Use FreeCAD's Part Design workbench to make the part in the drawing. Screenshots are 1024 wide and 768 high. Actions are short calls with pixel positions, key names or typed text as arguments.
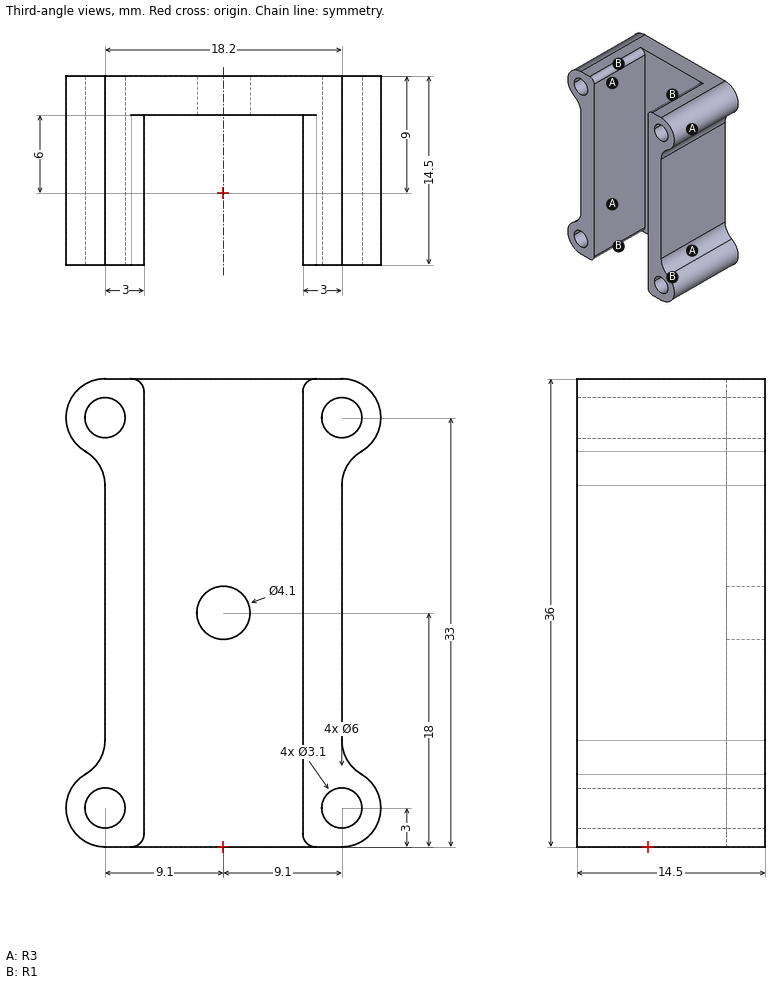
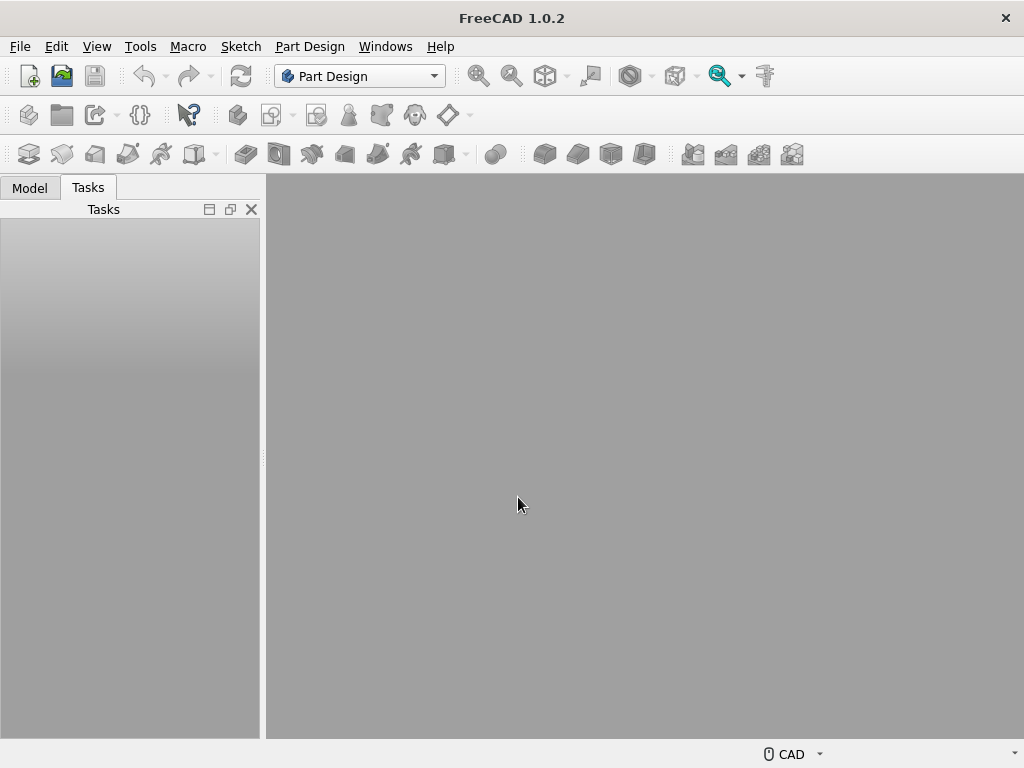
click(29, 76)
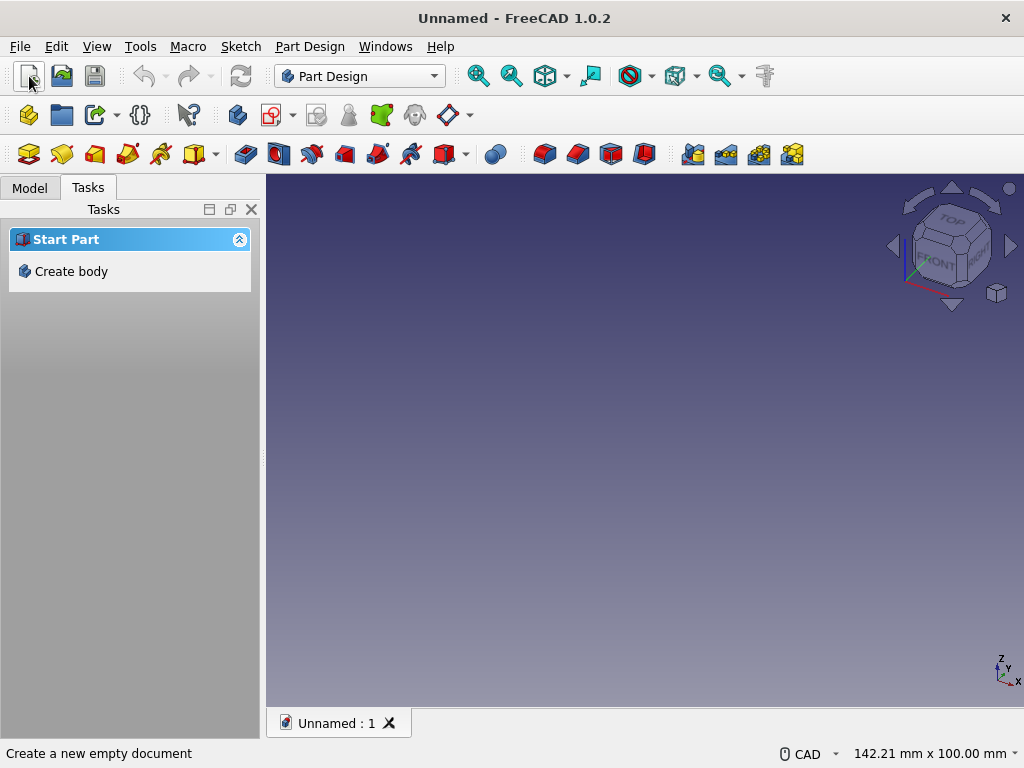
click(270, 116)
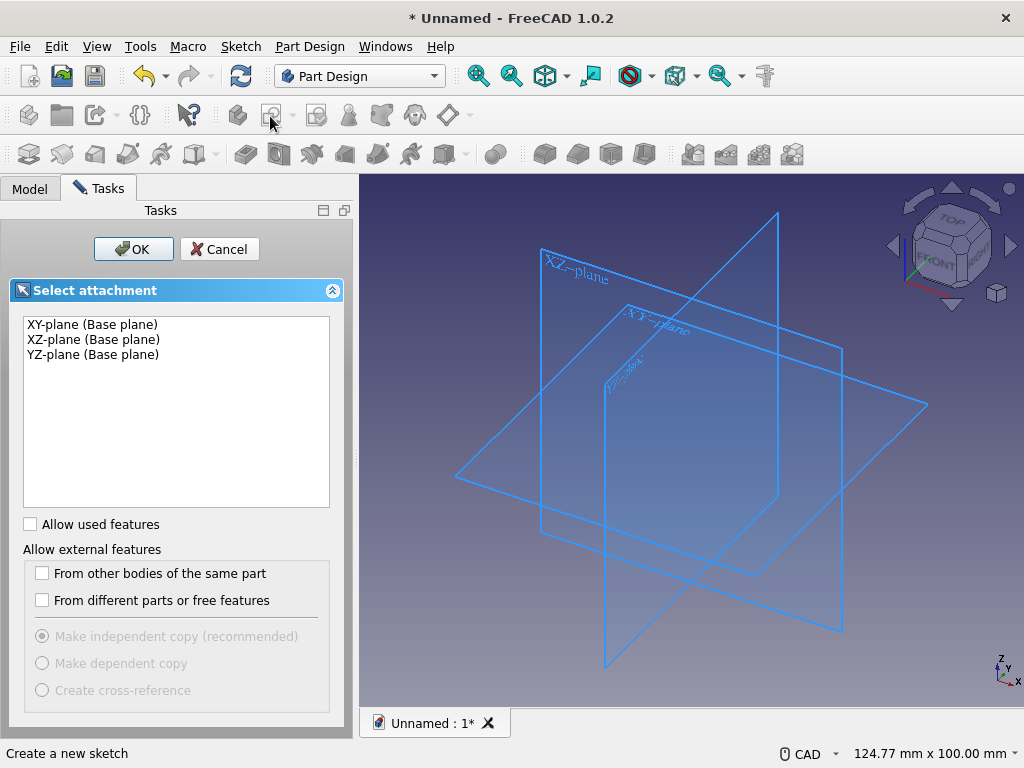
click(84, 324)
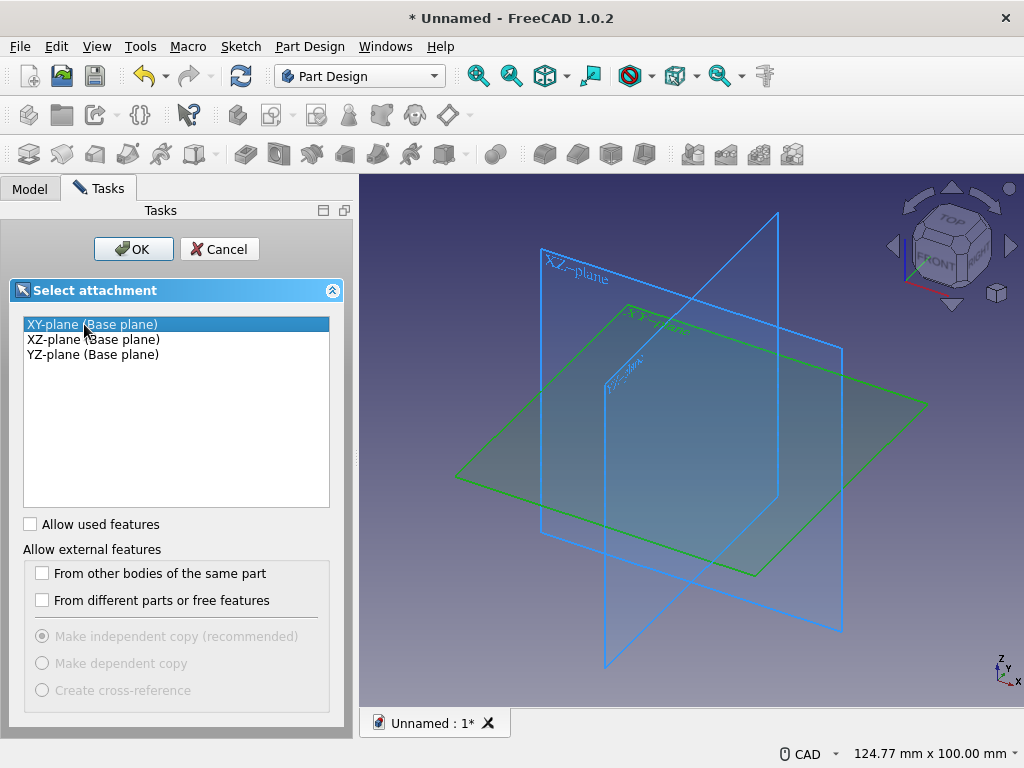
click(134, 249)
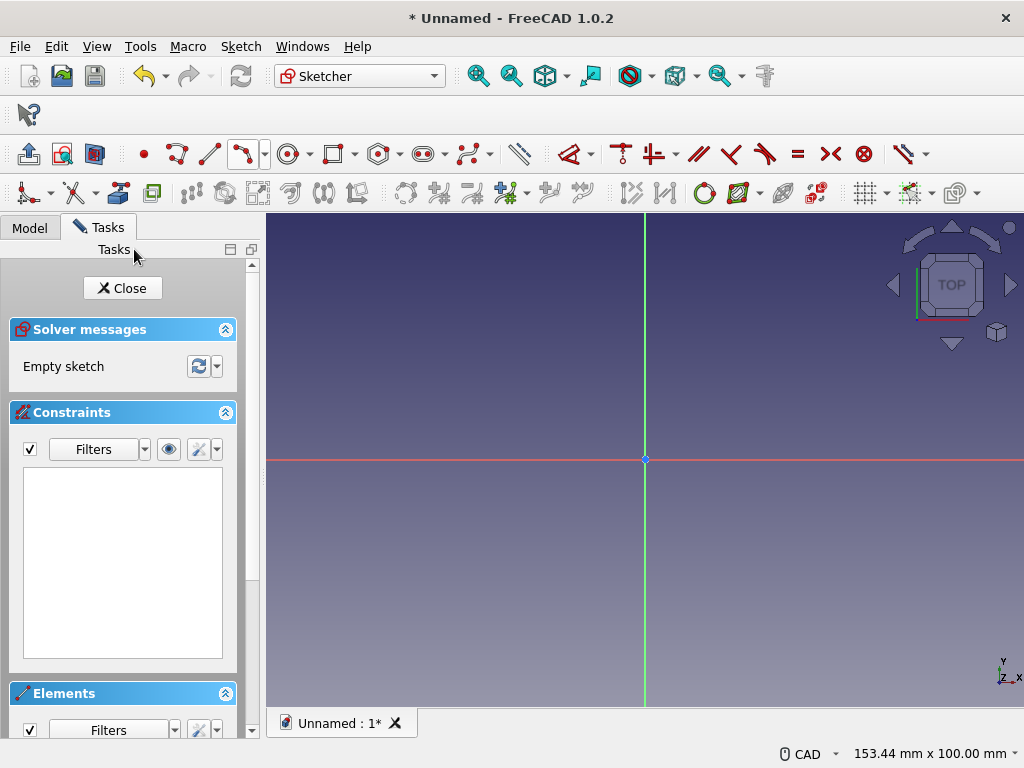
scroll(667, 449, up, 7)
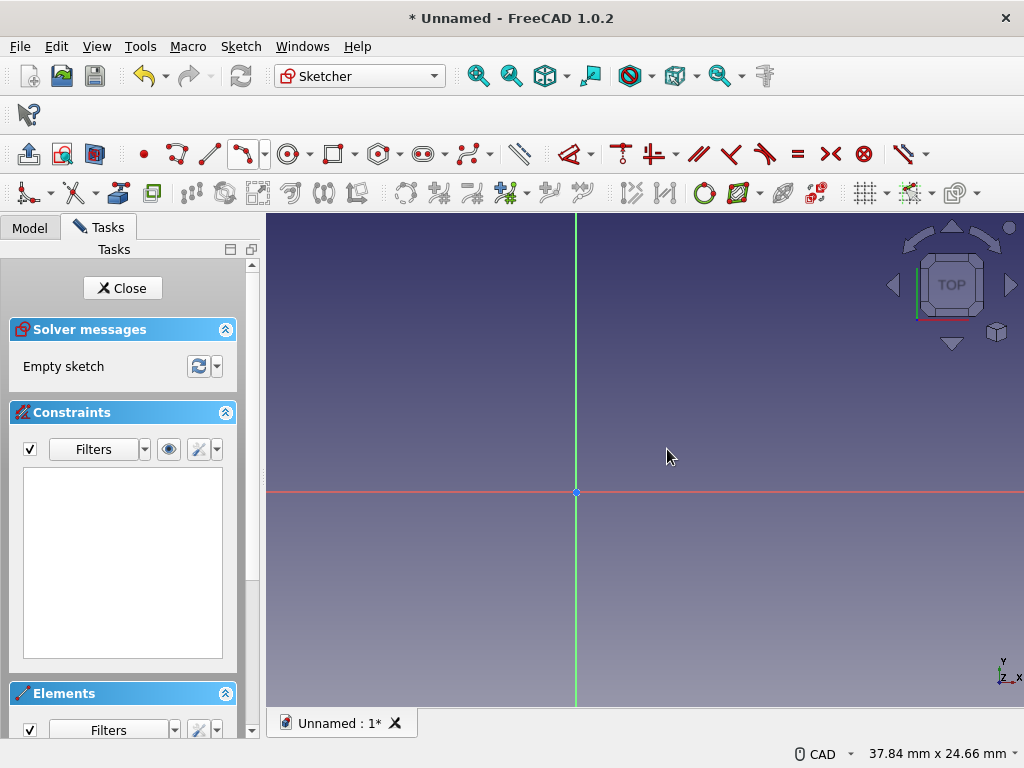
click(177, 154)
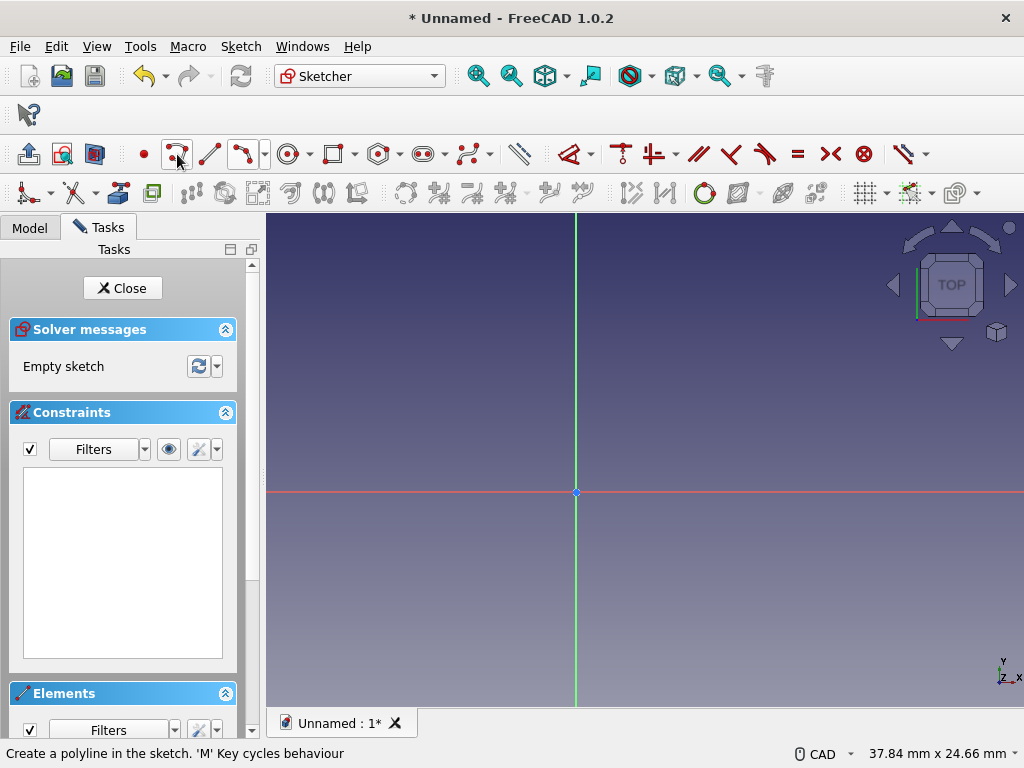
click(698, 602)
click(758, 602)
click(758, 312)
click(394, 312)
click(394, 602)
click(454, 602)
click(454, 372)
click(698, 372)
click(698, 603)
key(Escape)
key(Escape)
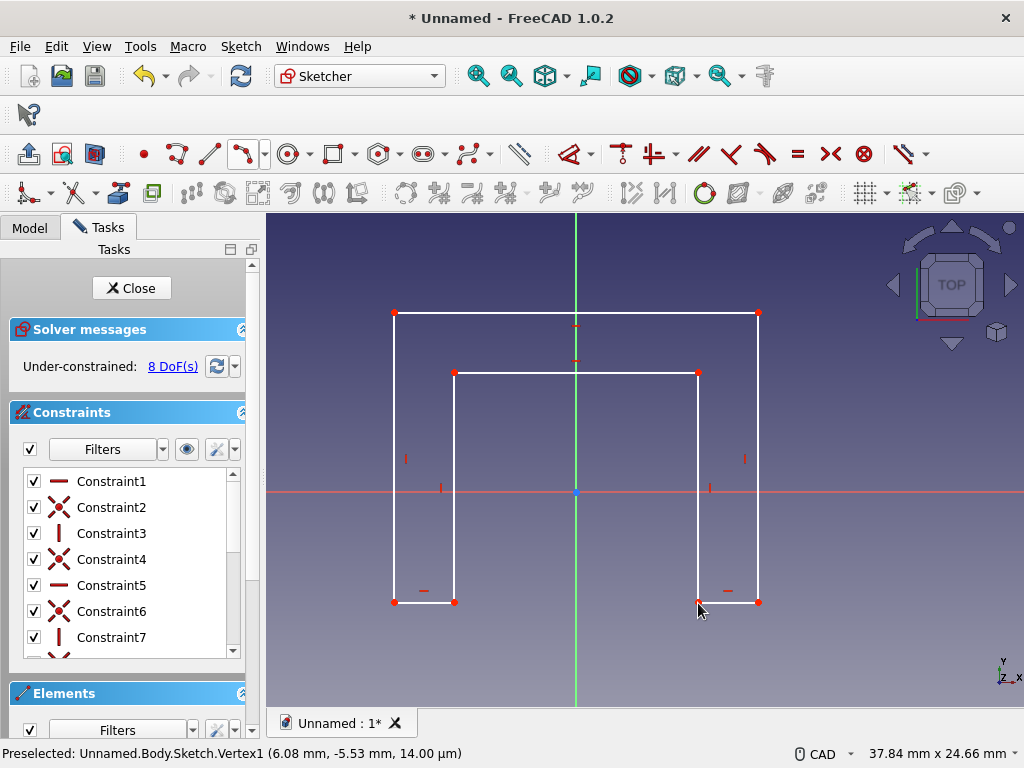
click(758, 603)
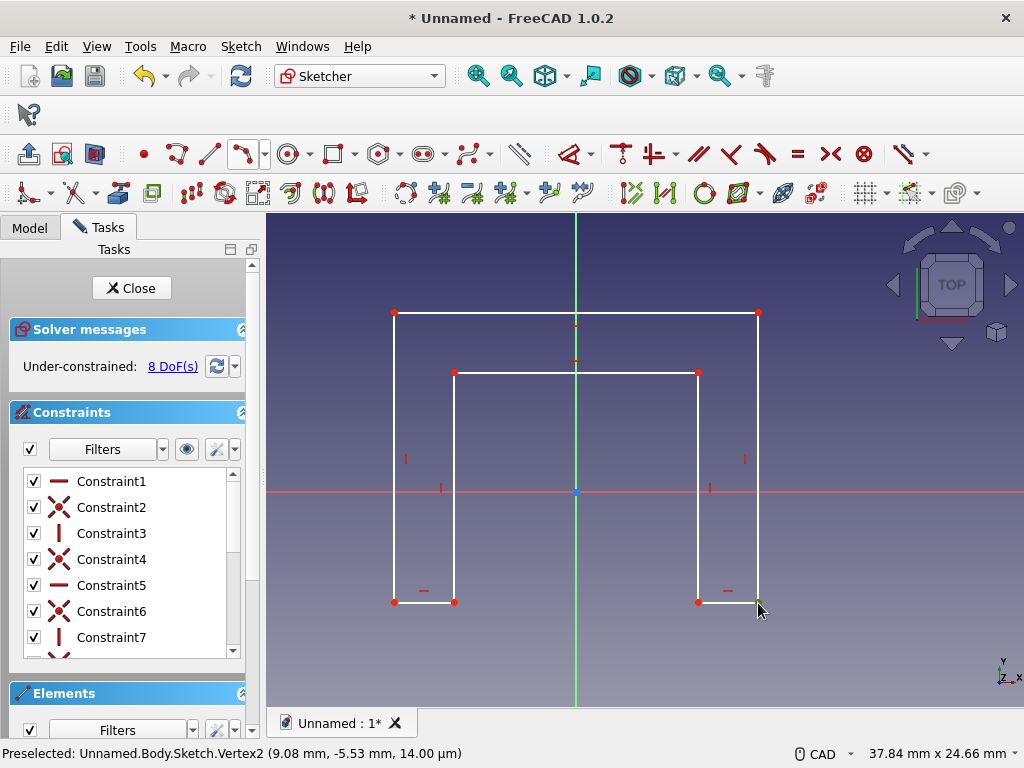
click(394, 603)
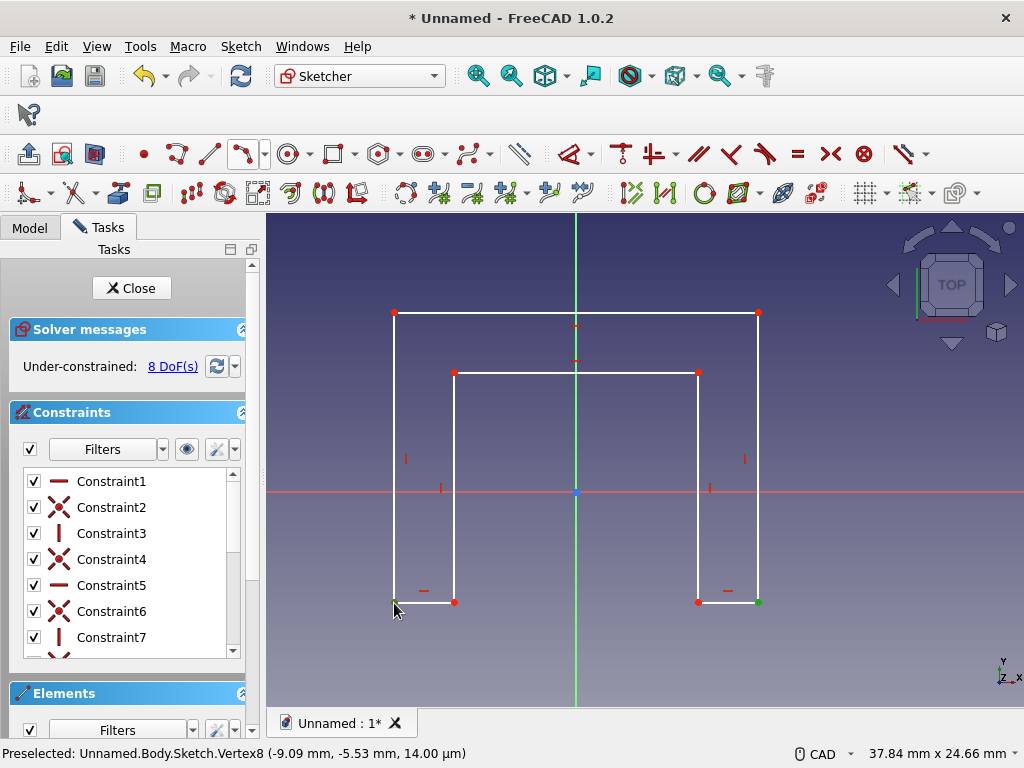
click(576, 648)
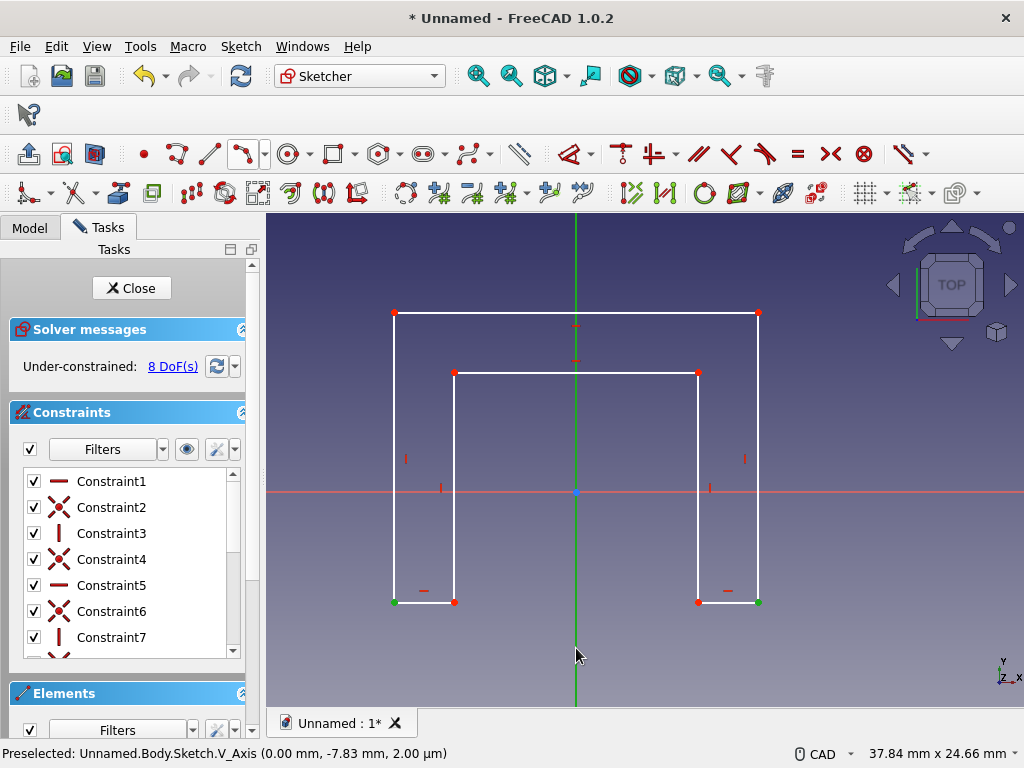
click(831, 154)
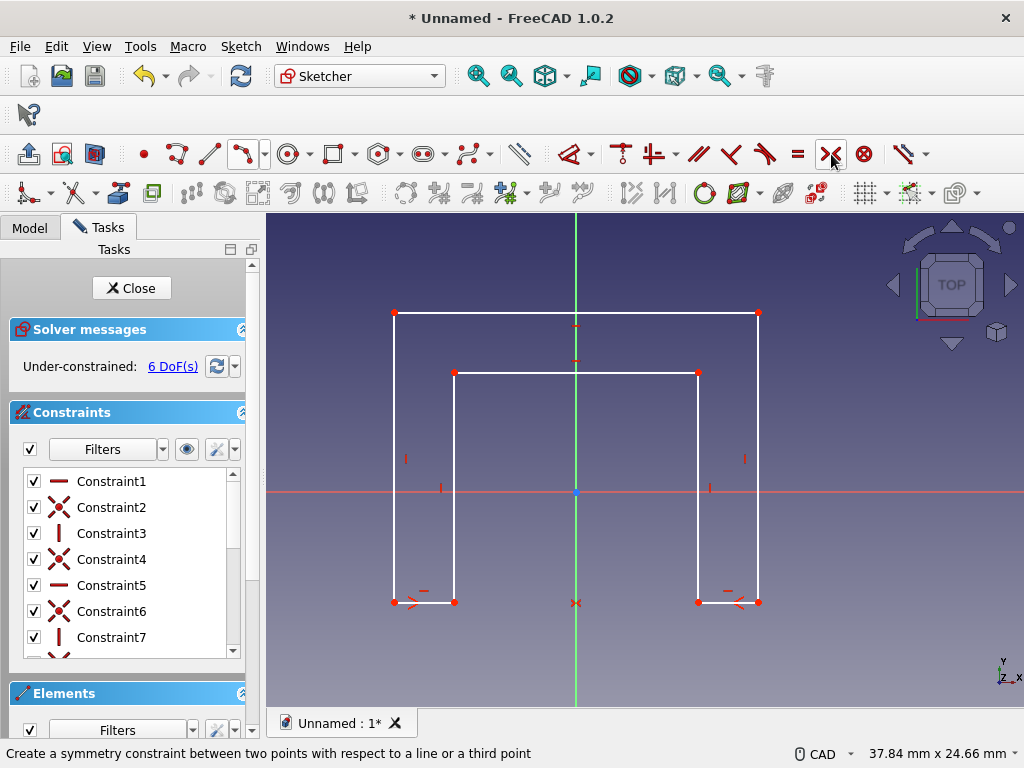
click(568, 154)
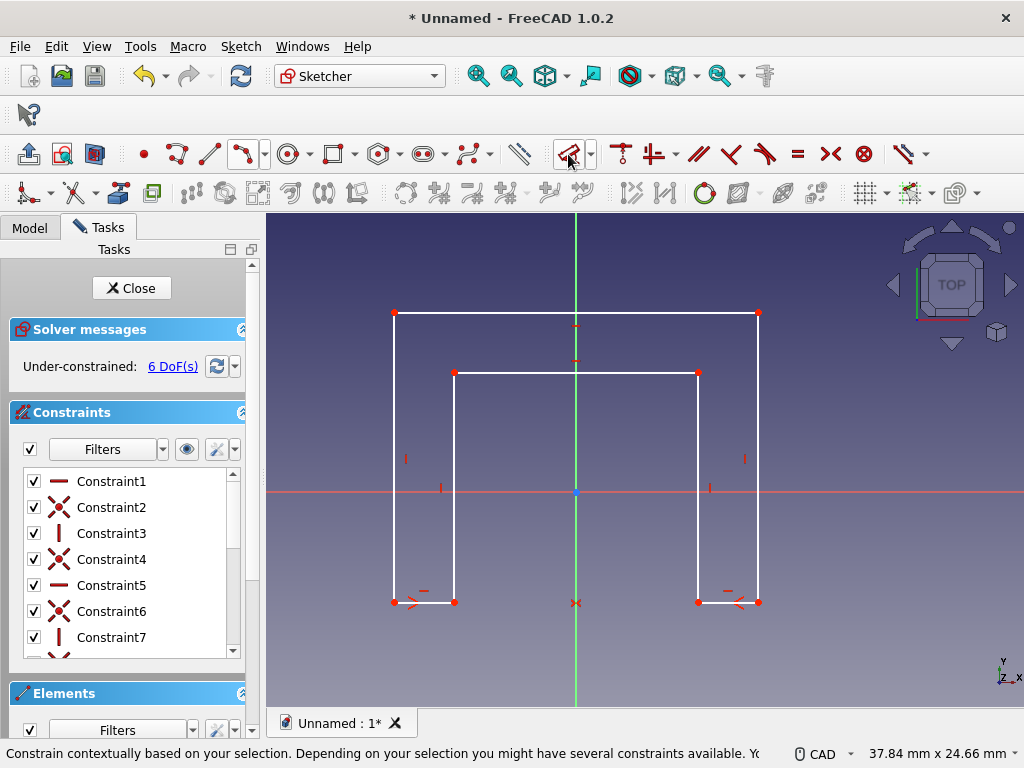
click(716, 603)
click(728, 637)